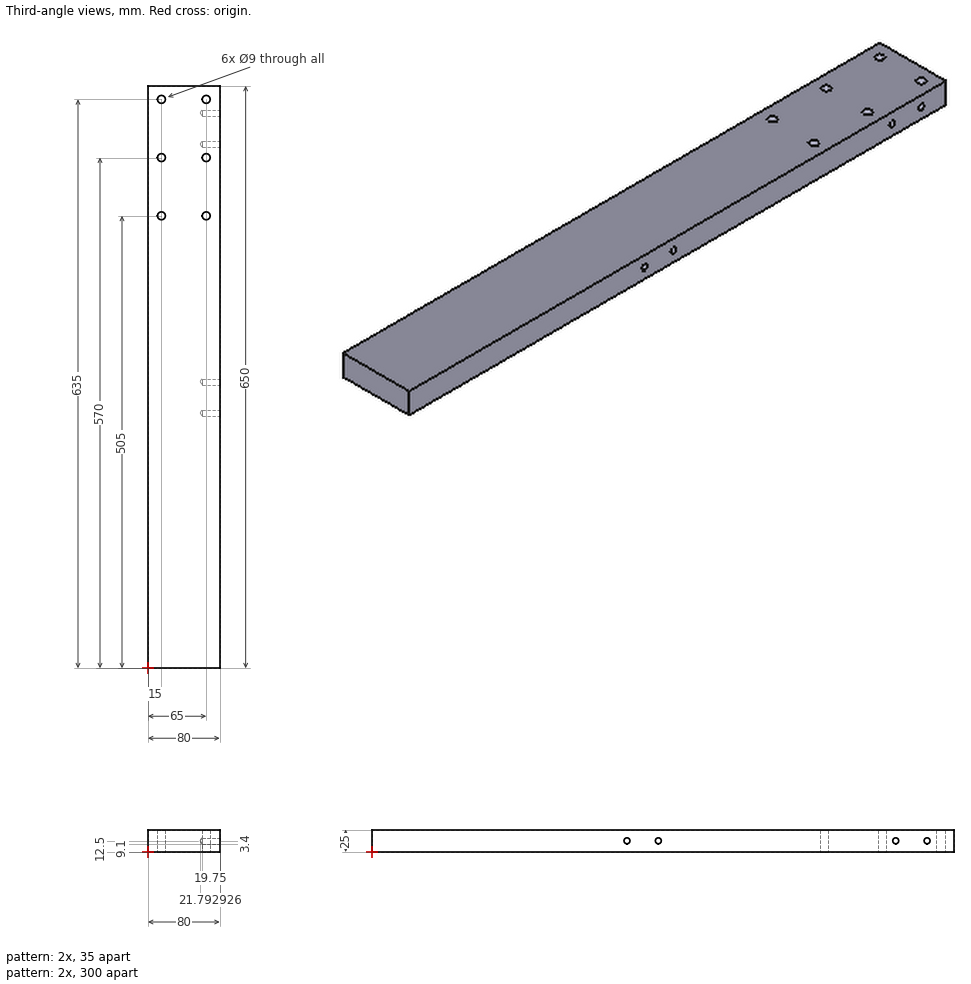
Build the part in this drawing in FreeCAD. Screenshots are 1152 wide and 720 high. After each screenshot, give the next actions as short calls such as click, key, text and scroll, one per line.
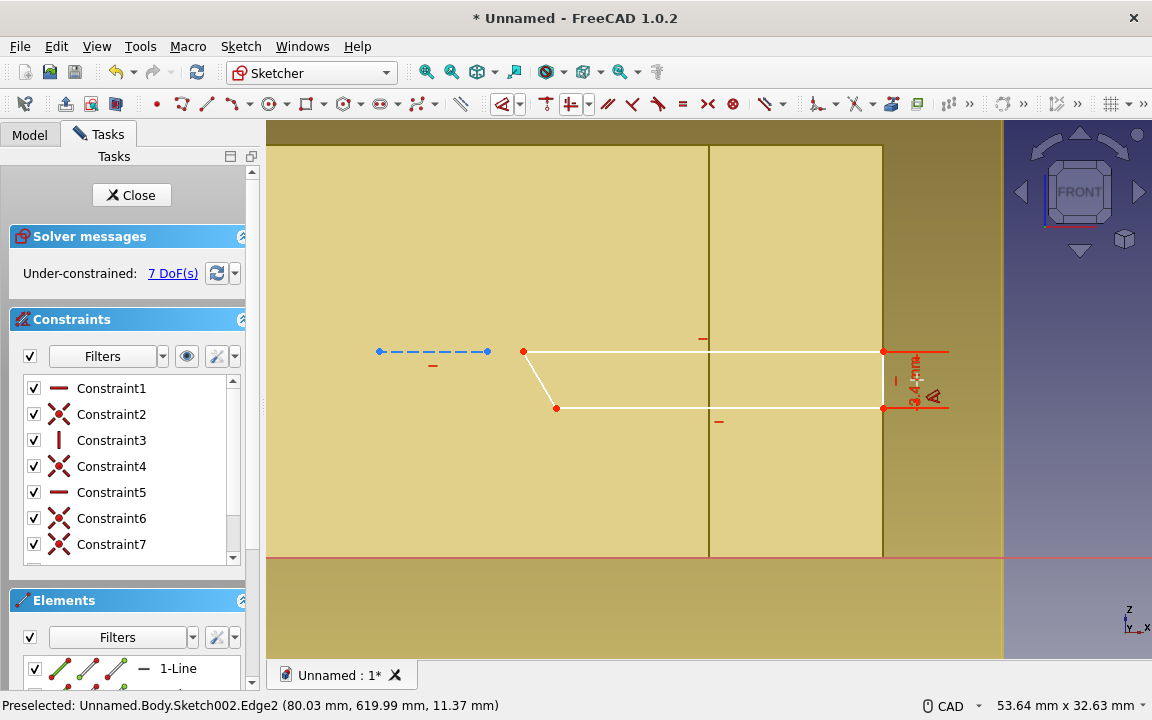
click(883, 352)
click(588, 592)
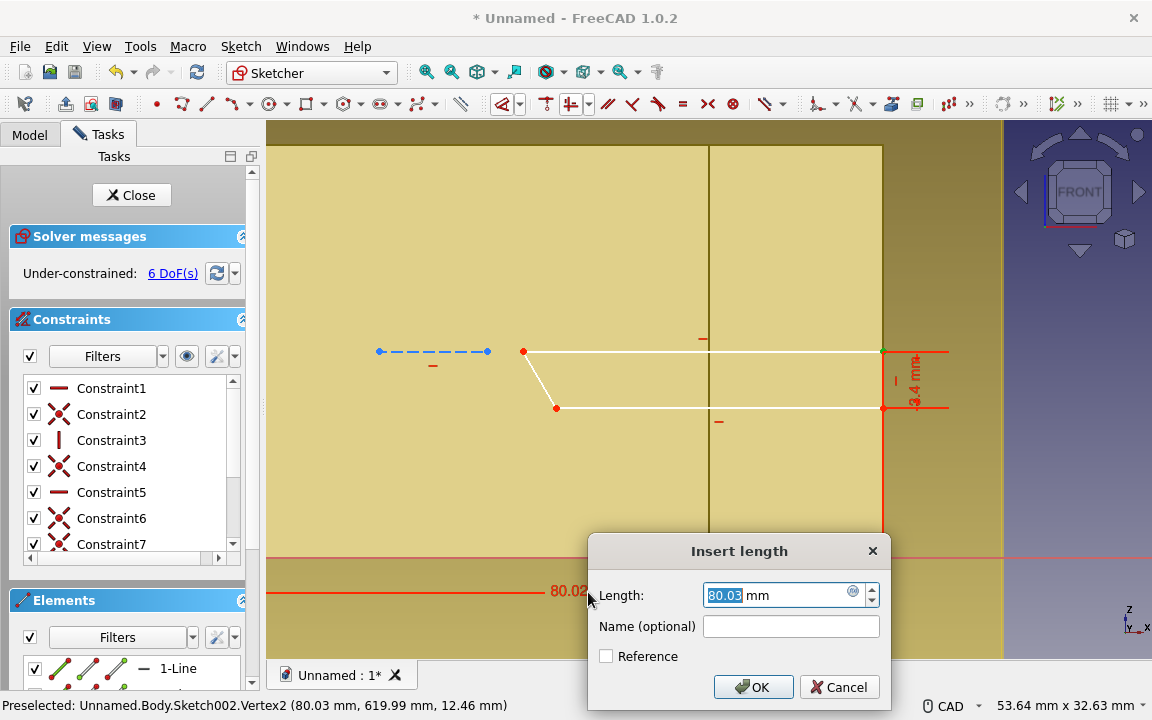
text(80)
key(Return)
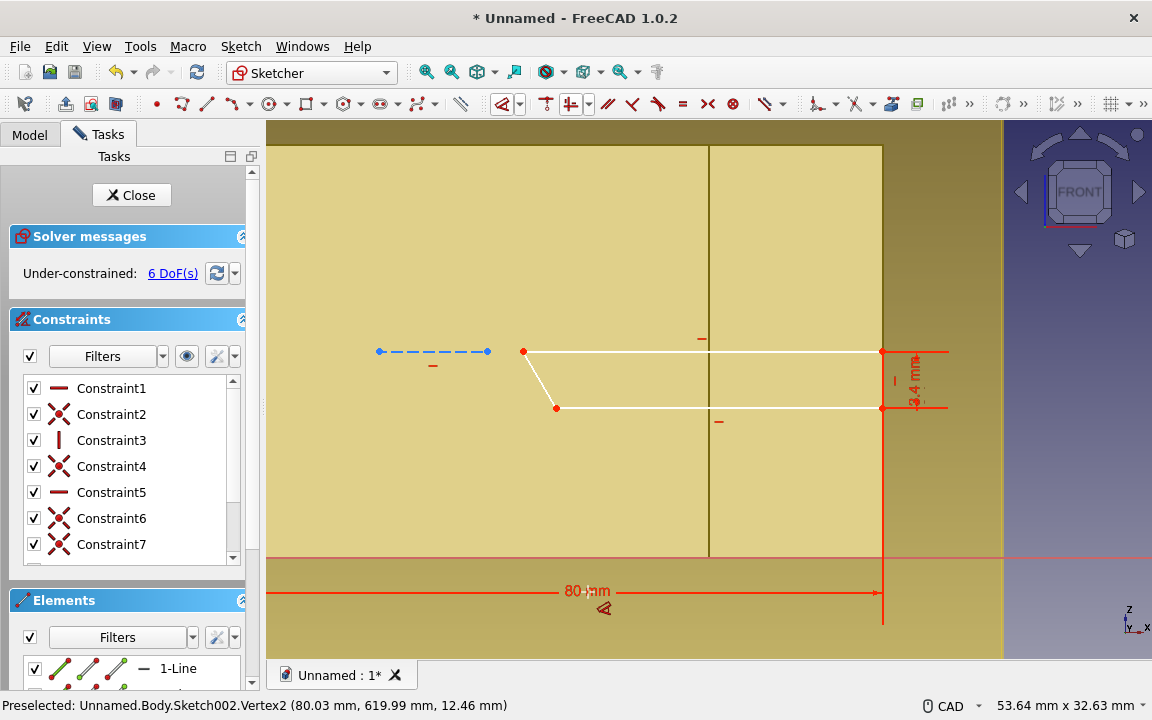
click(883, 408)
click(917, 483)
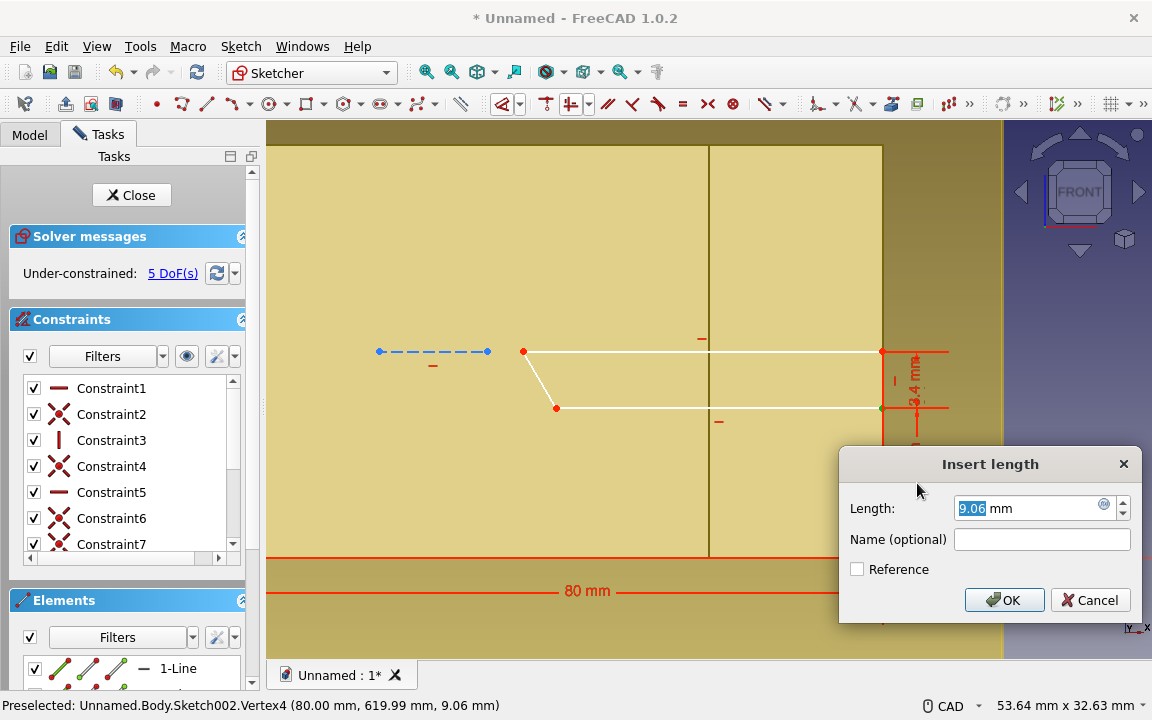
text(9.1)
key(Return)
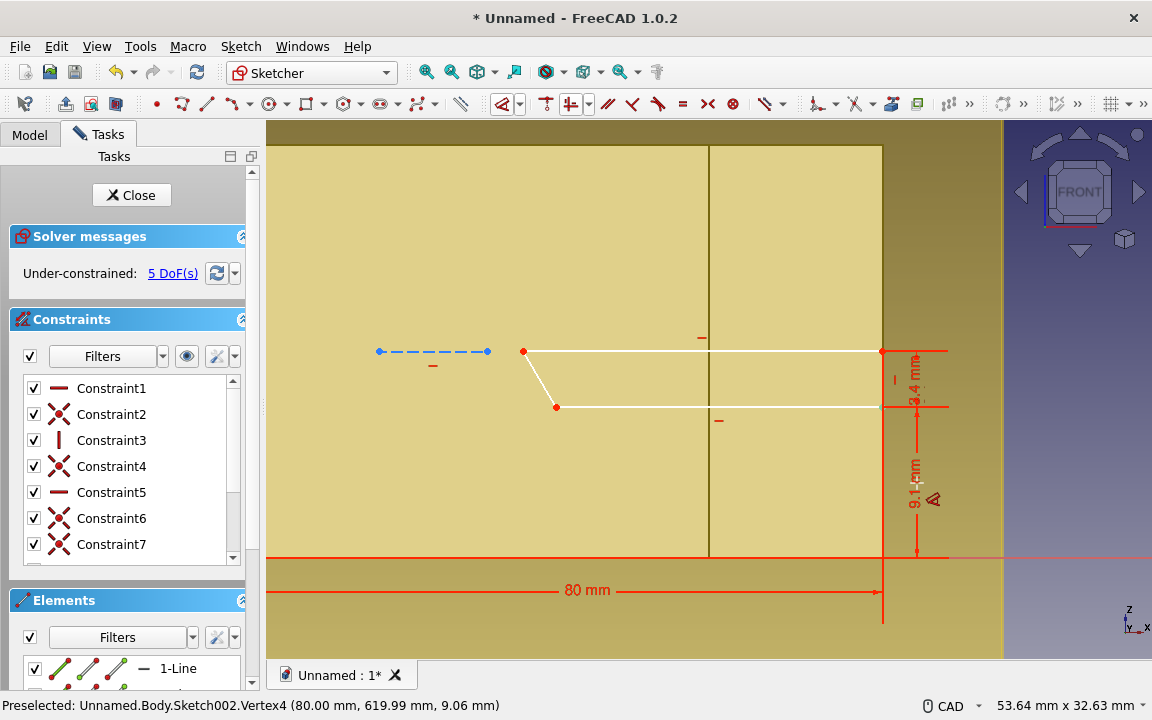
click(785, 407)
click(719, 441)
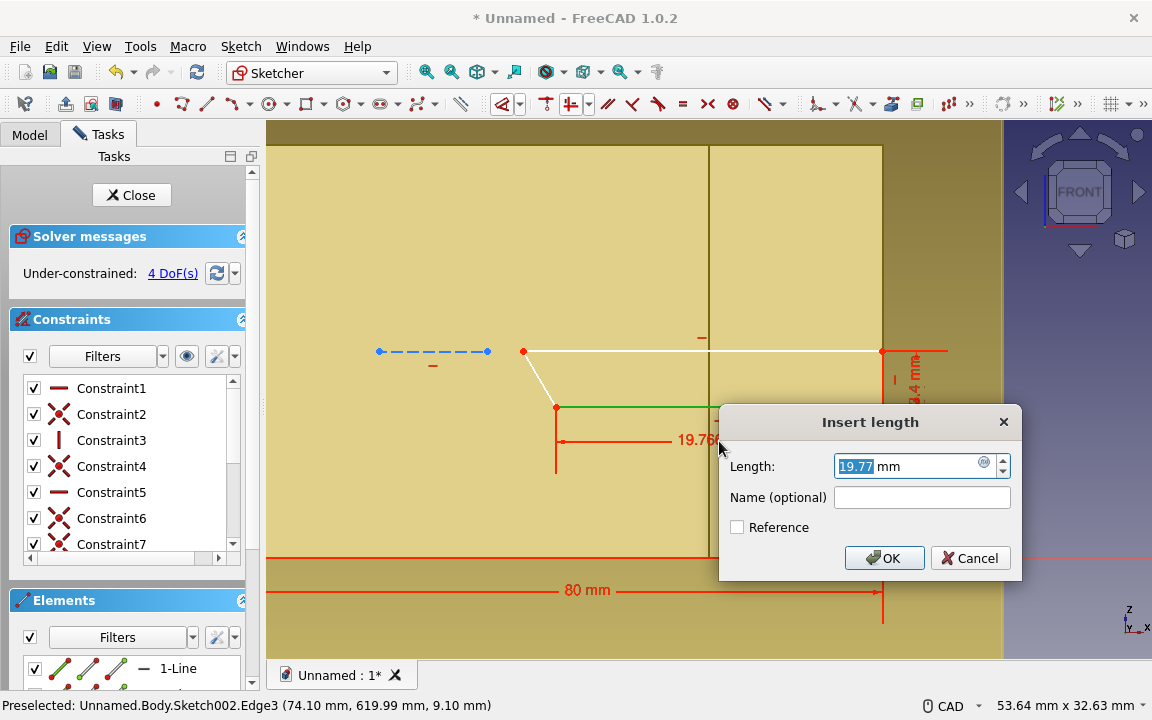
text(19.75)
key(Return)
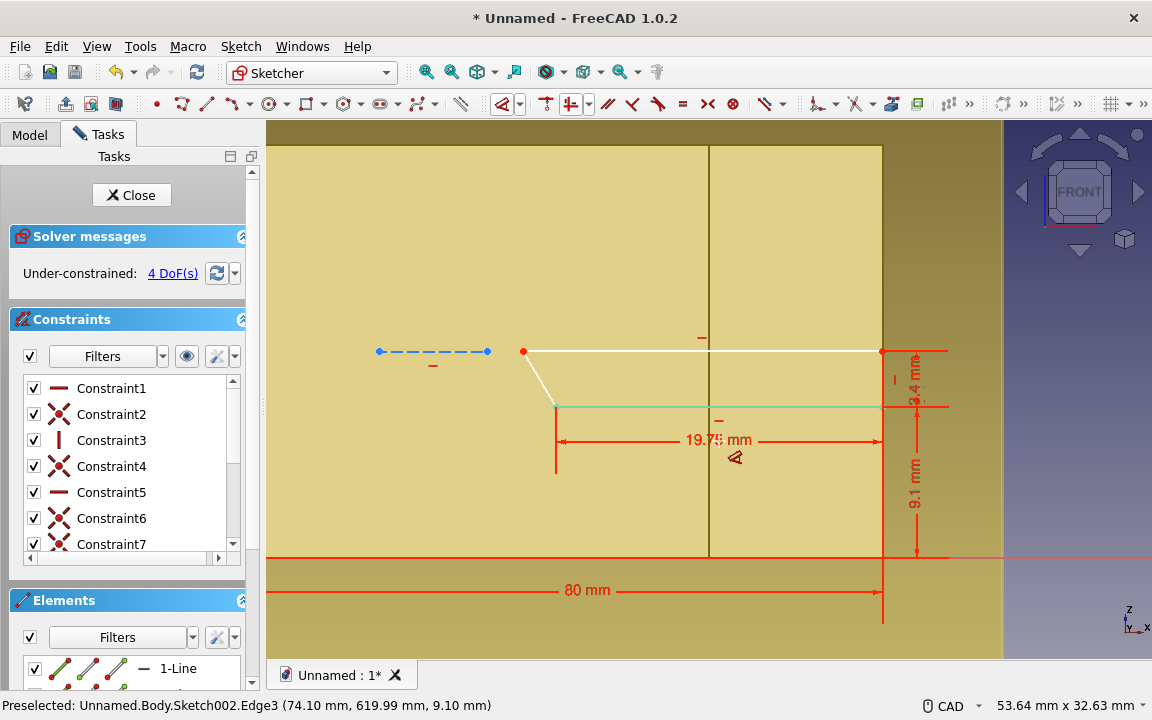
click(487, 352)
click(521, 455)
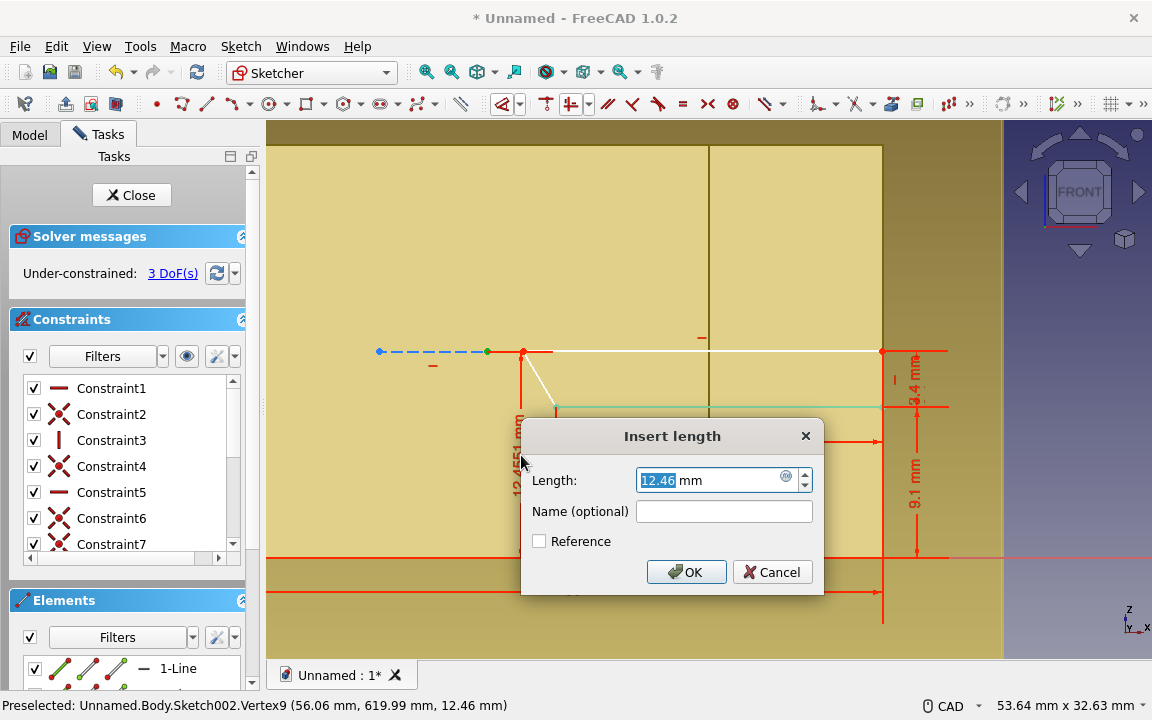
text(12.5)
key(Return)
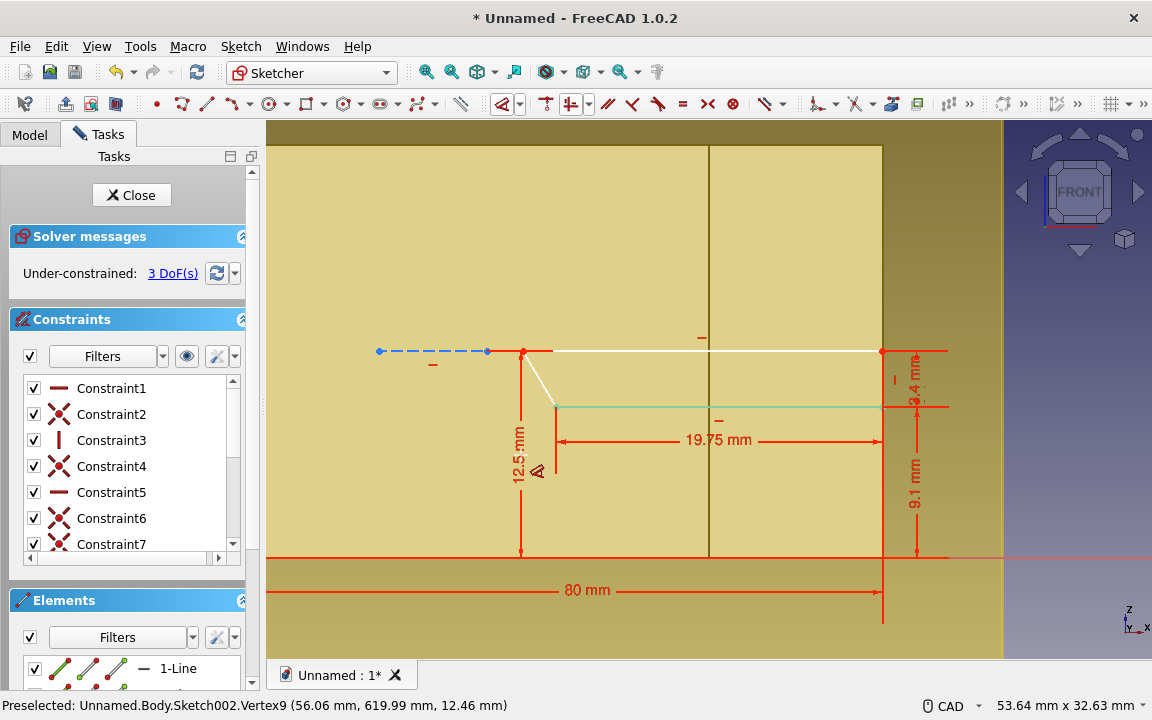
click(631, 351)
click(703, 317)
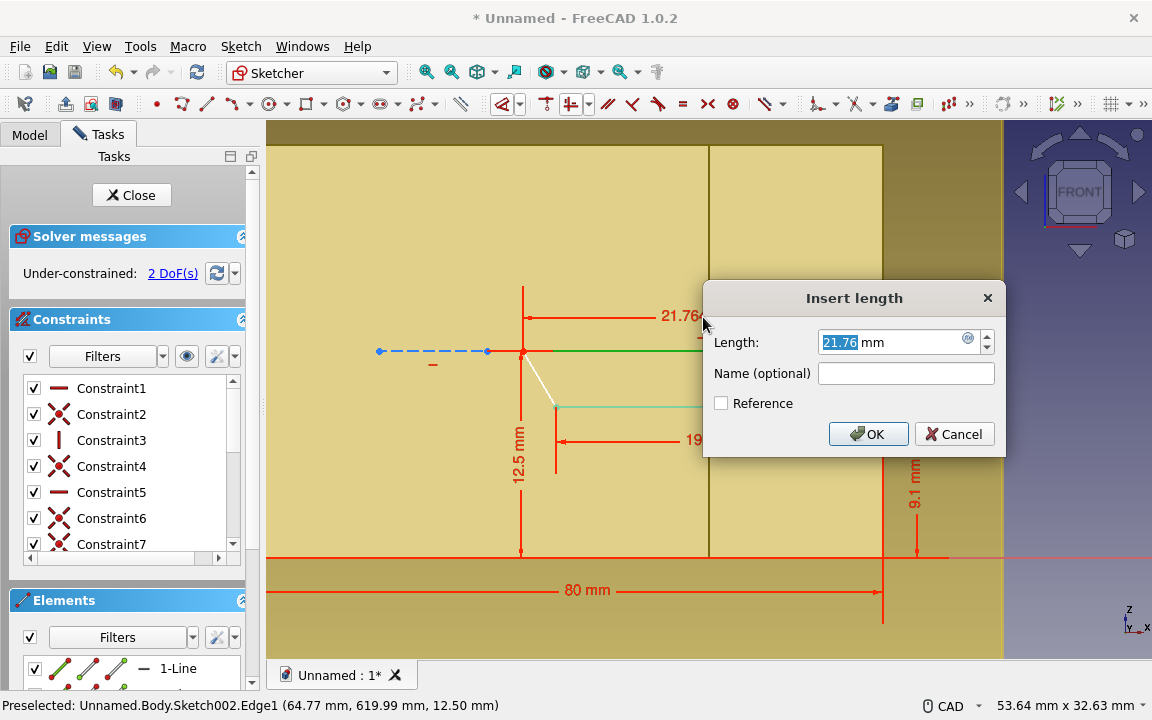
text(21.792926)
key(Return)
key(Escape)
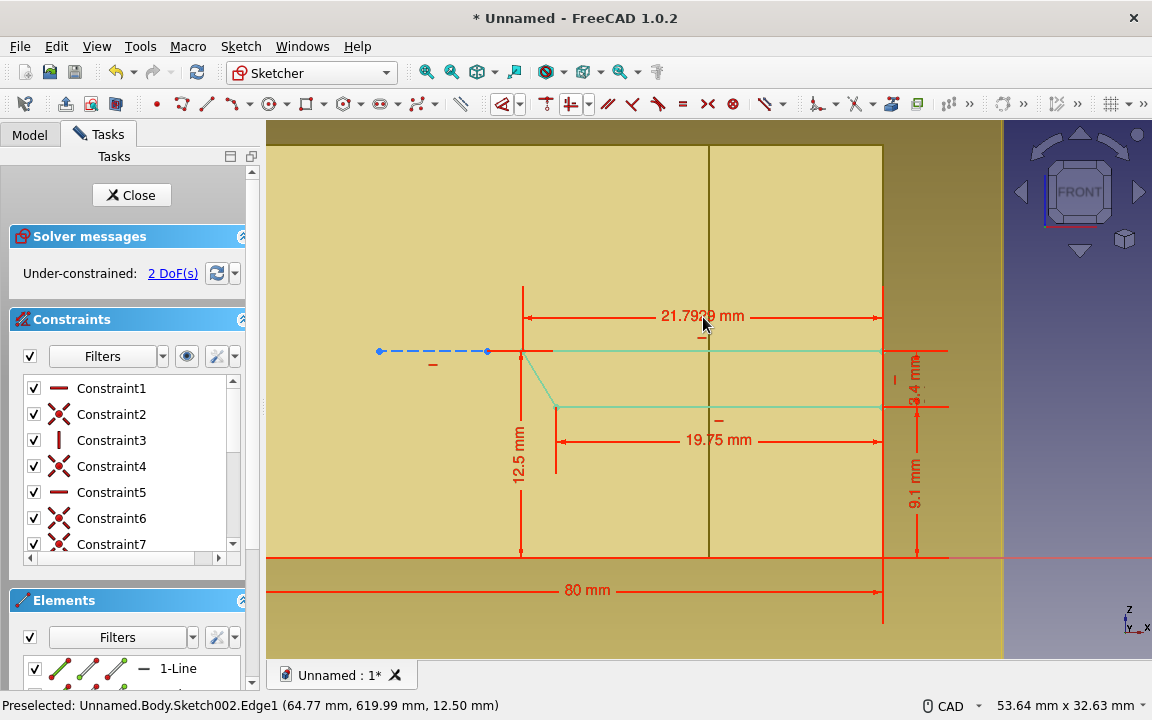
click(132, 195)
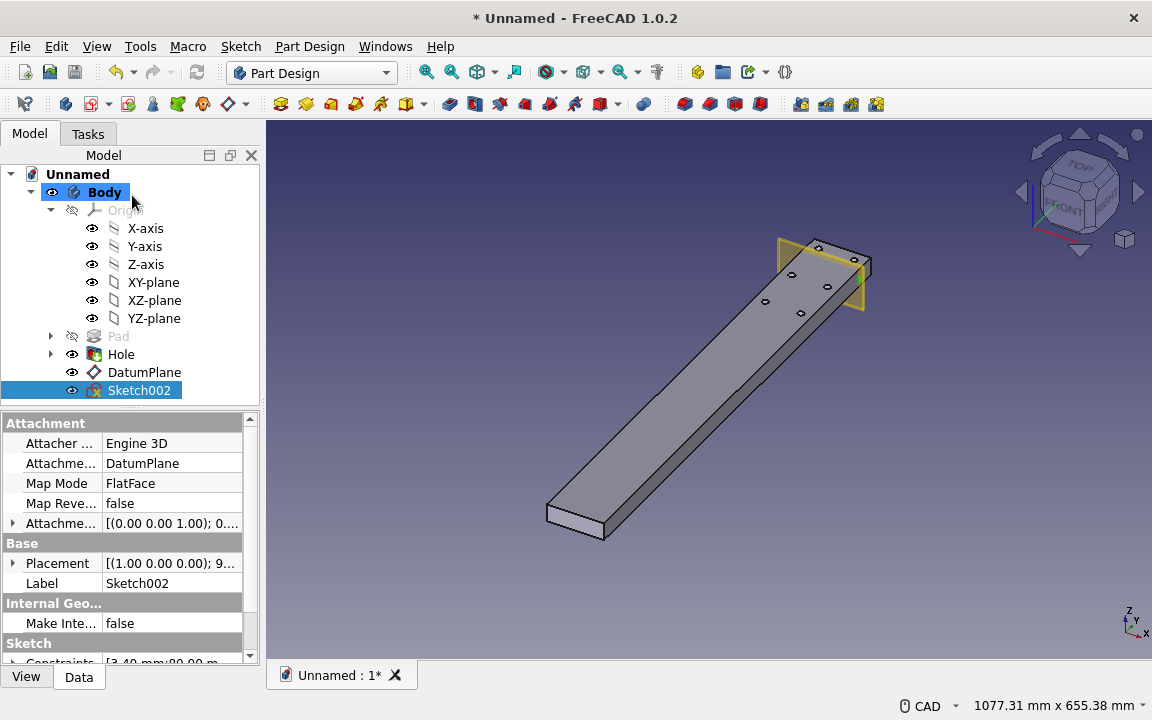
click(500, 104)